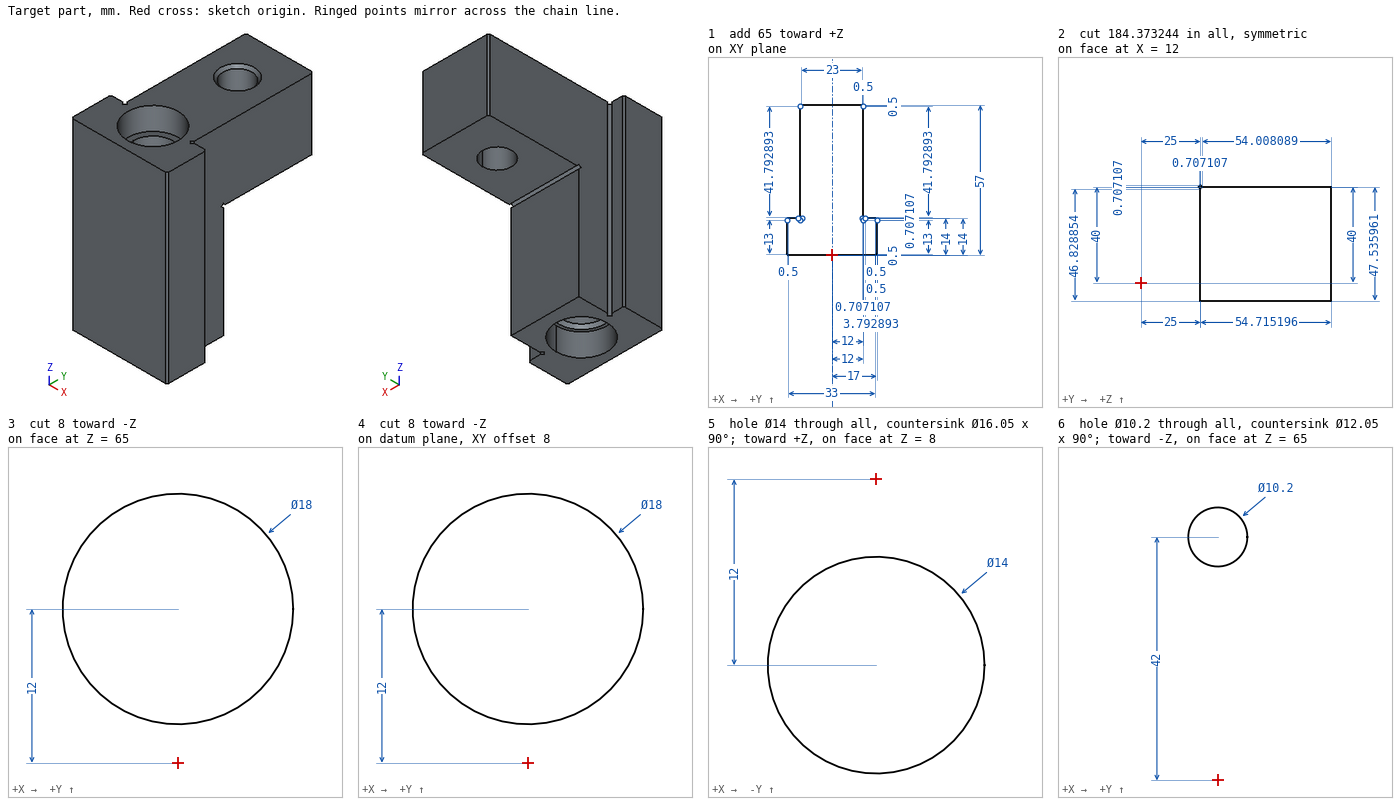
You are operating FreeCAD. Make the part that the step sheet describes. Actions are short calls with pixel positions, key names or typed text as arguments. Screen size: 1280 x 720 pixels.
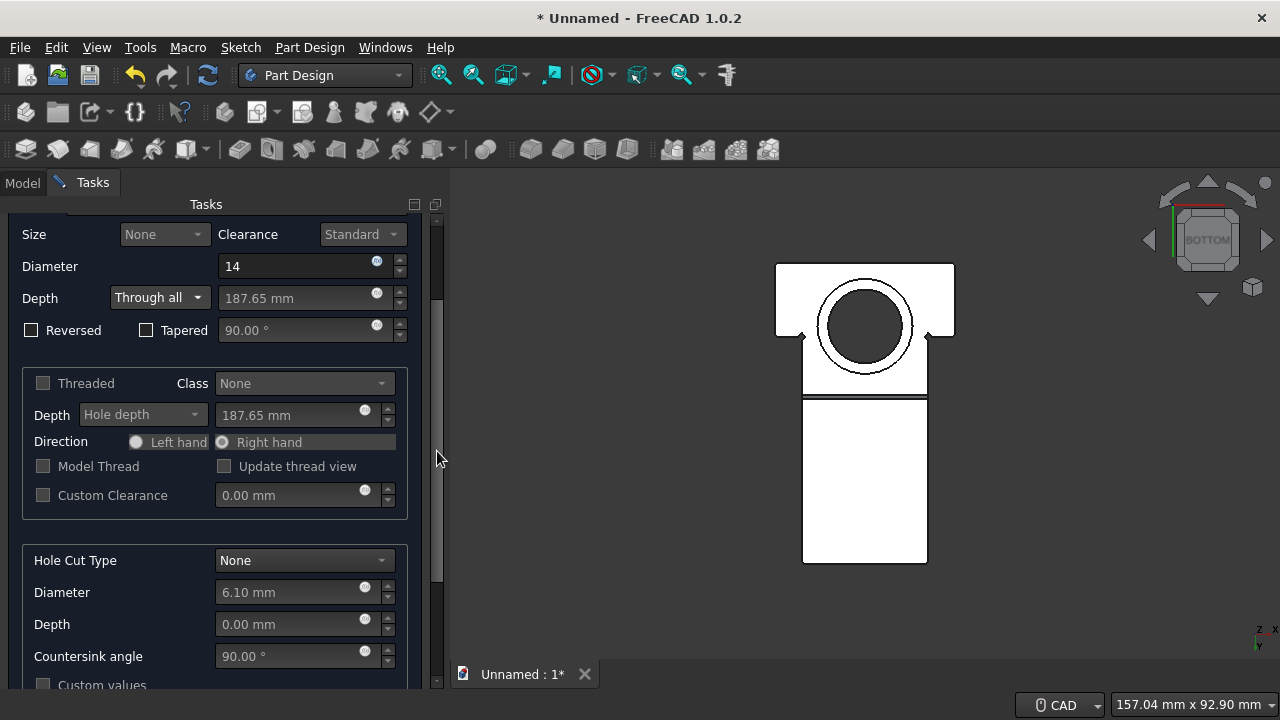
click(306, 560)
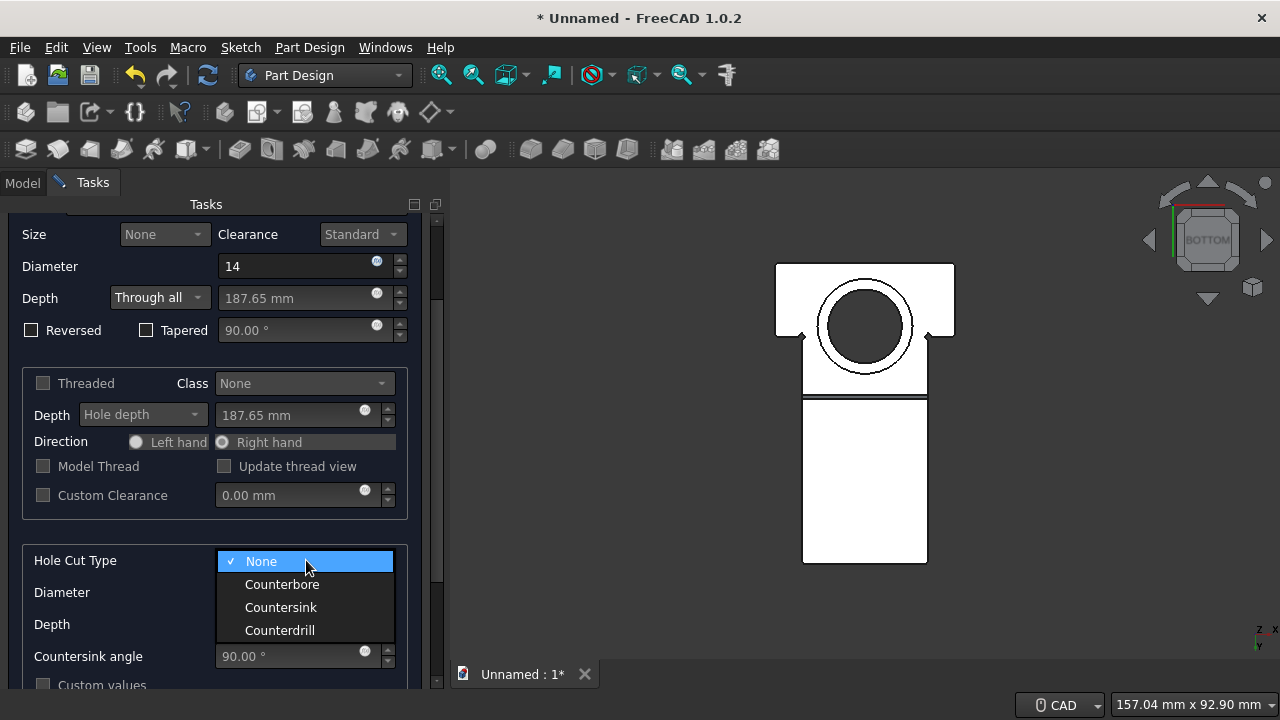
click(304, 608)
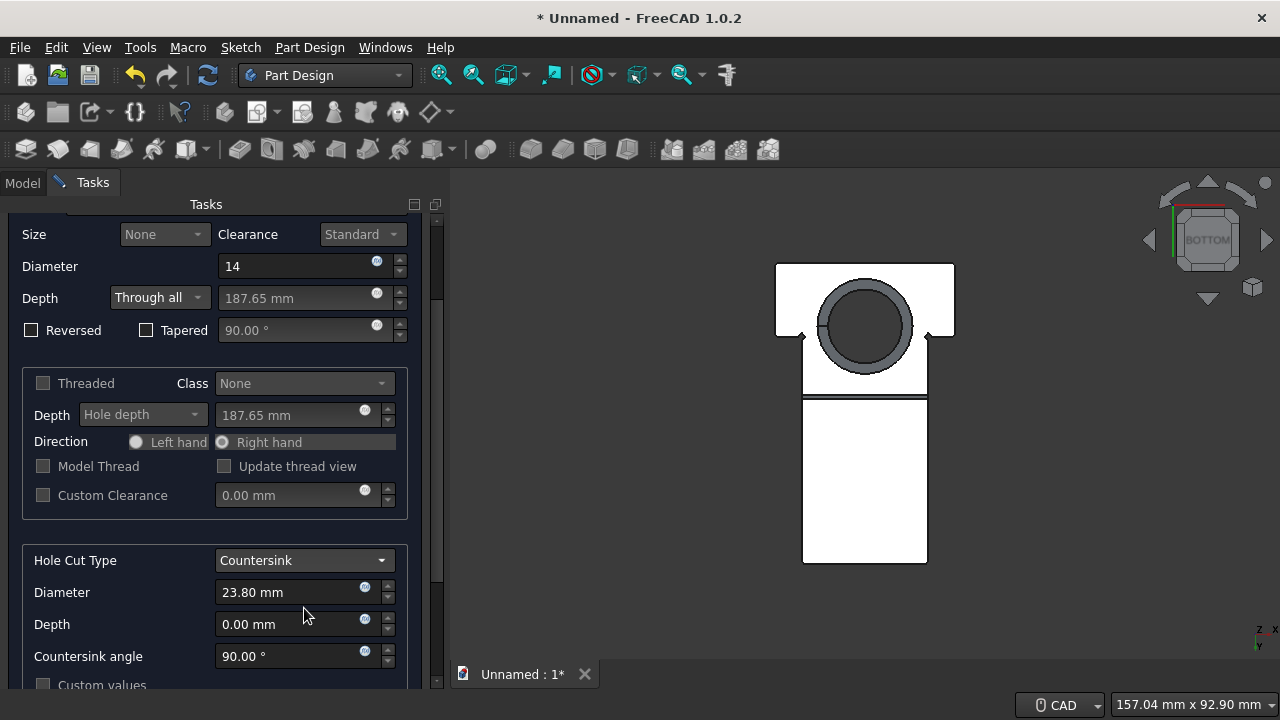
triple_click(298, 592)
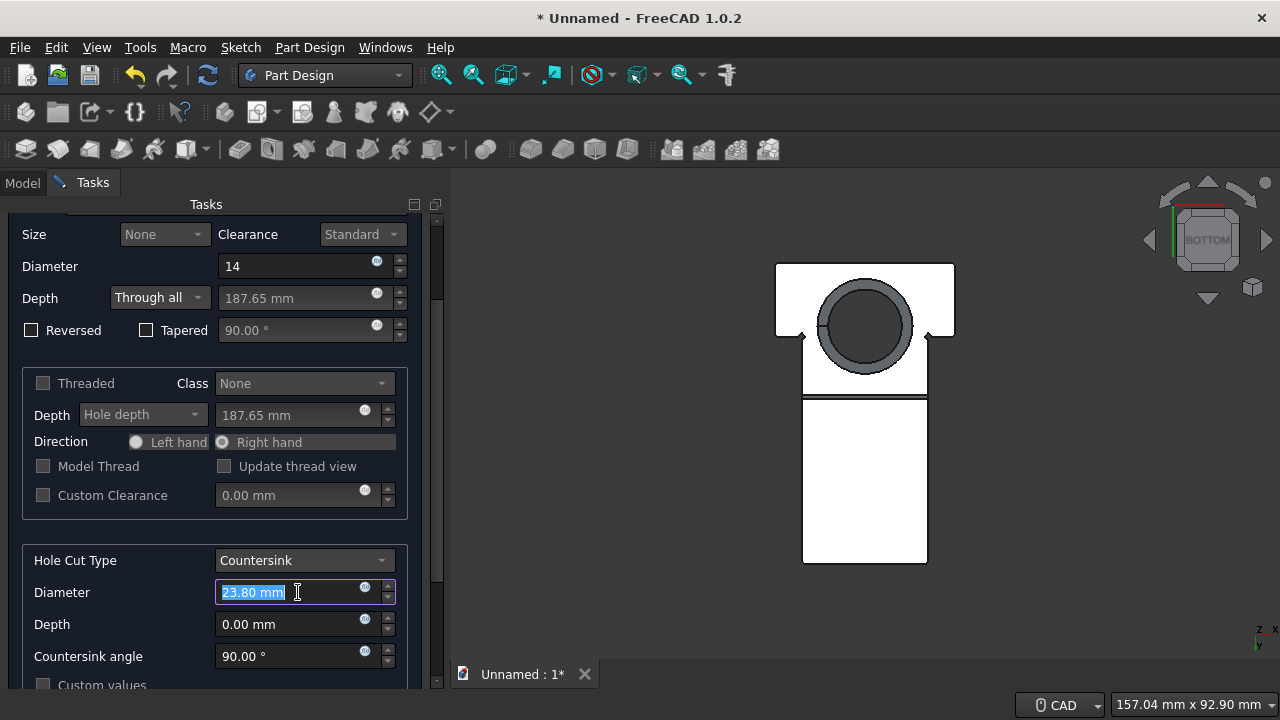
text(16.05)
key(Tab)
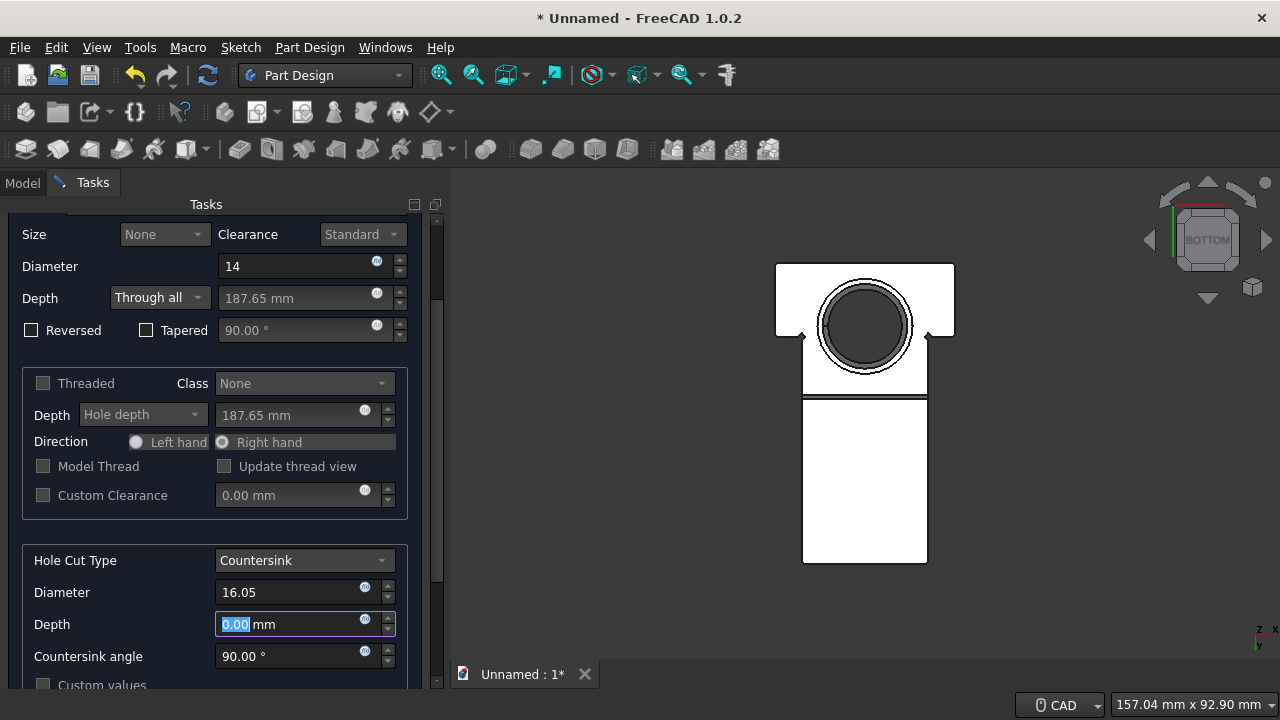
scroll(437, 451, up, 3)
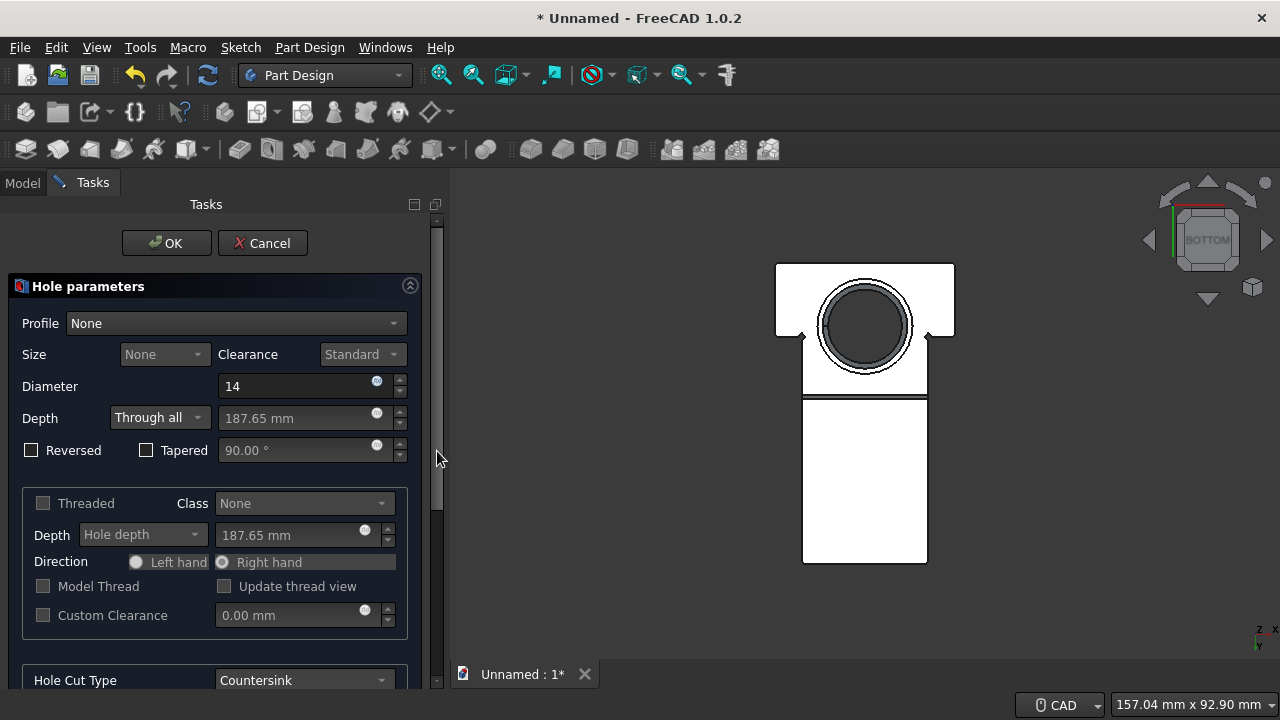
click(167, 243)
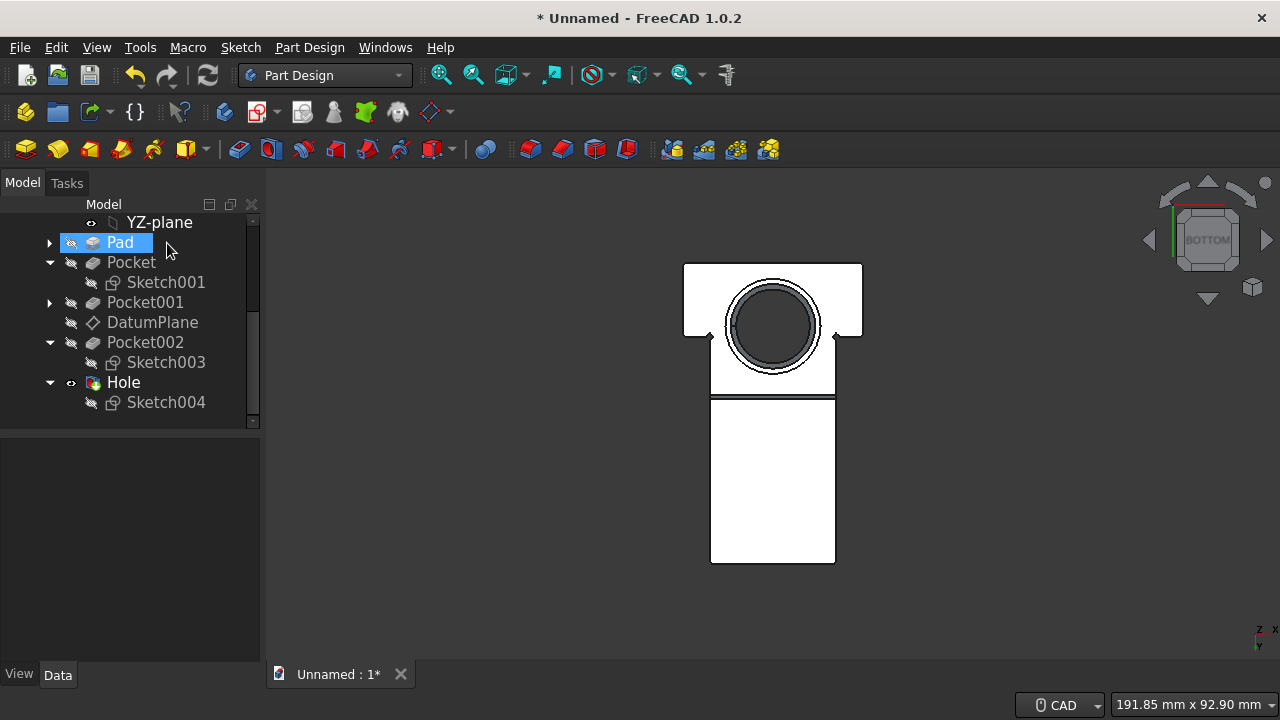
key(0)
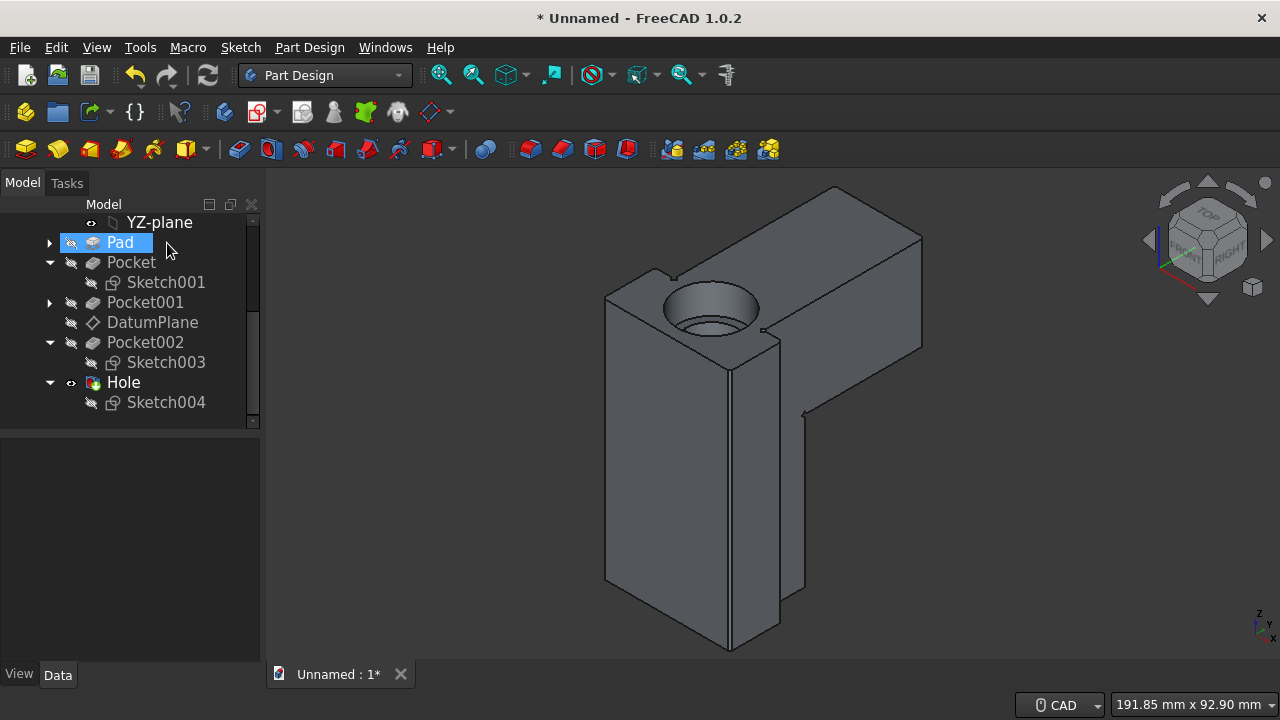
click(834, 237)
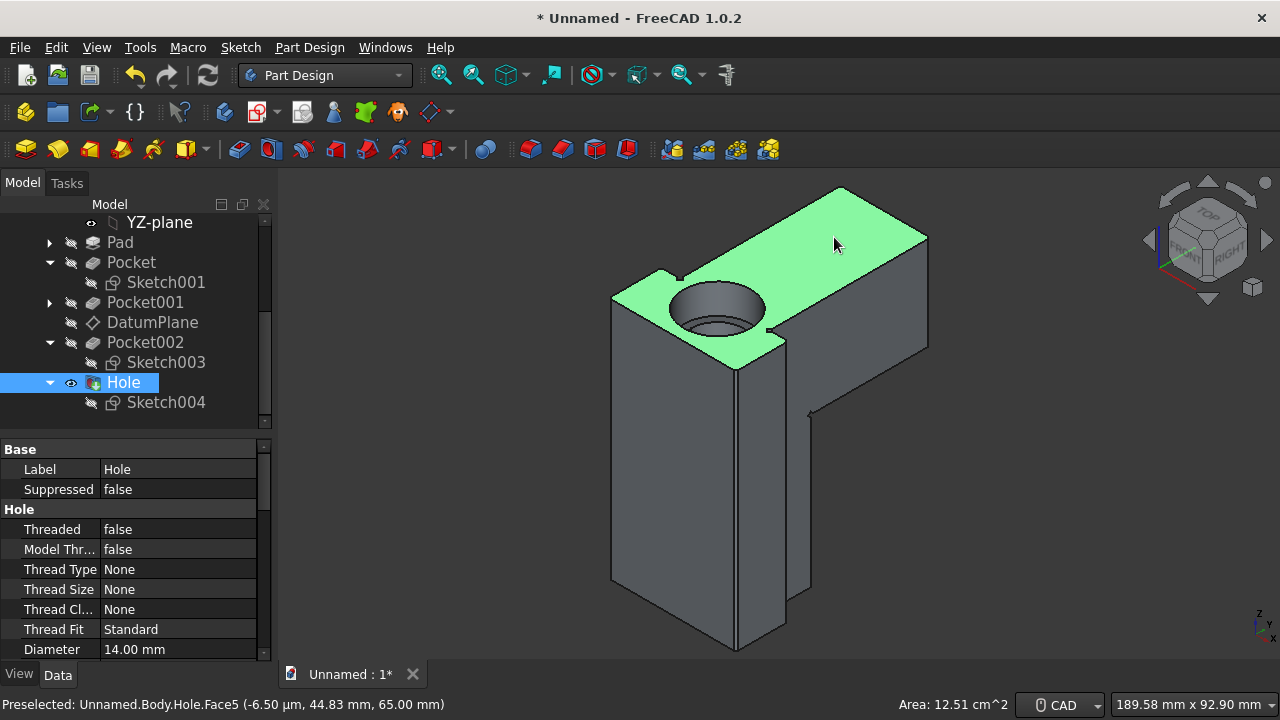
click(258, 112)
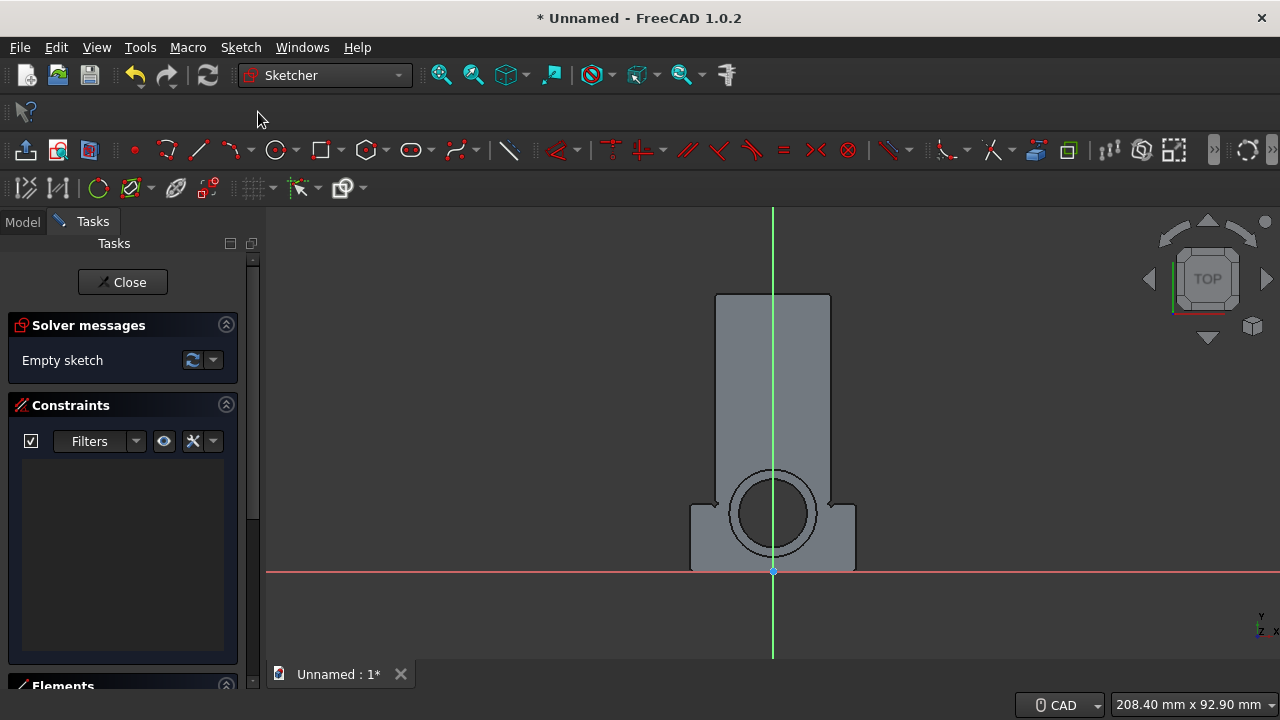
scroll(787, 354, up, 9)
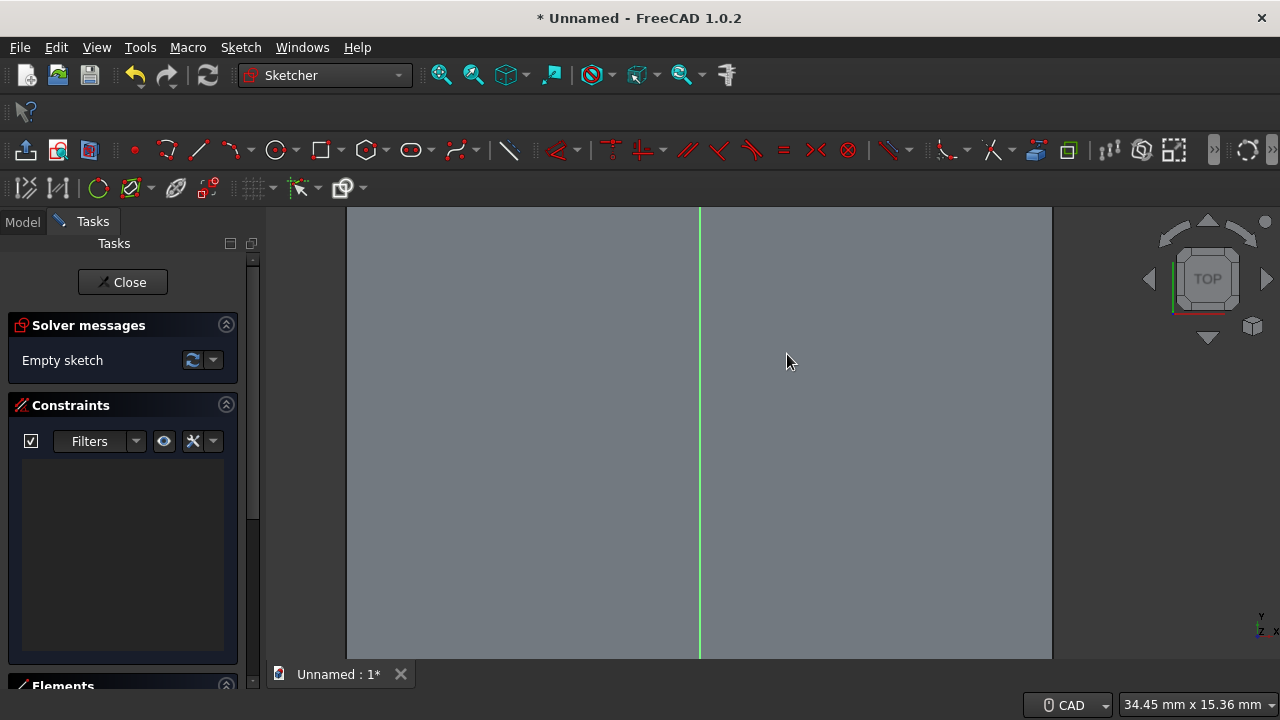
click(276, 150)